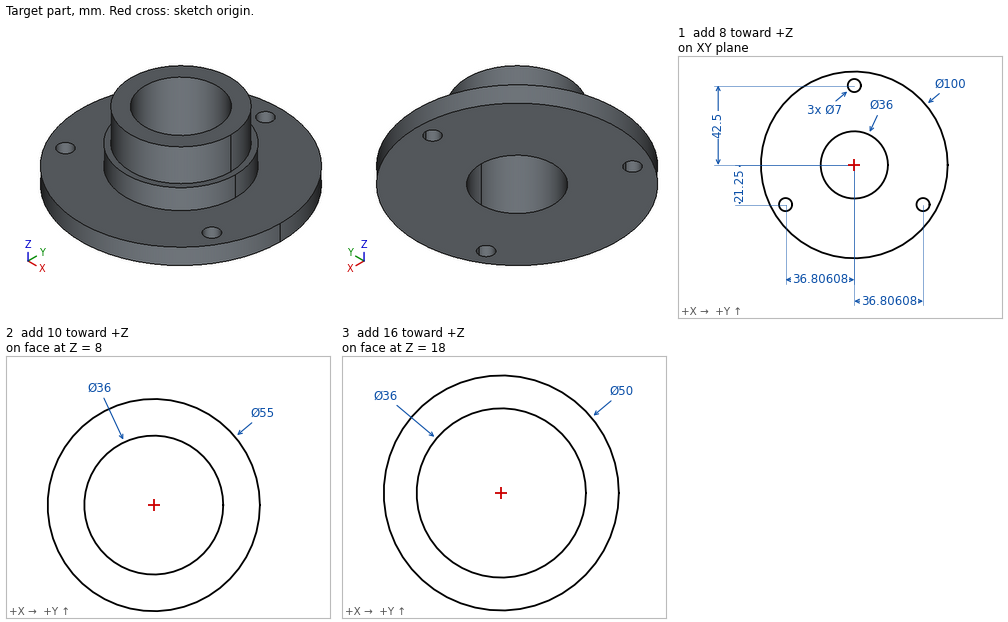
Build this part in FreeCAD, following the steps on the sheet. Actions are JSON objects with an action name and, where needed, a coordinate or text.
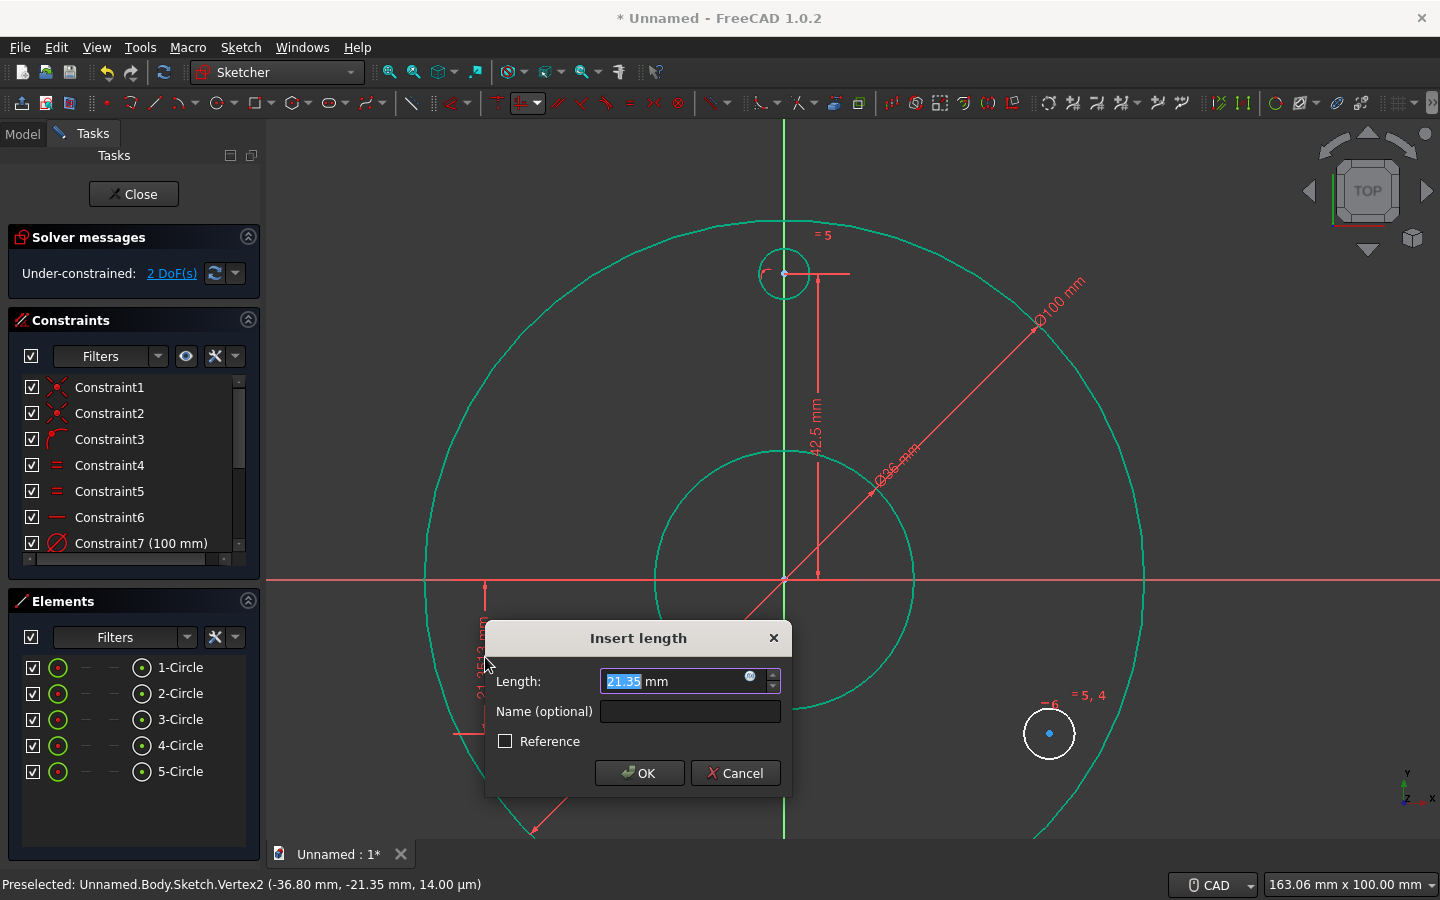
{"action": "type", "text": "21.25"}
{"action": "key", "text": "Return"}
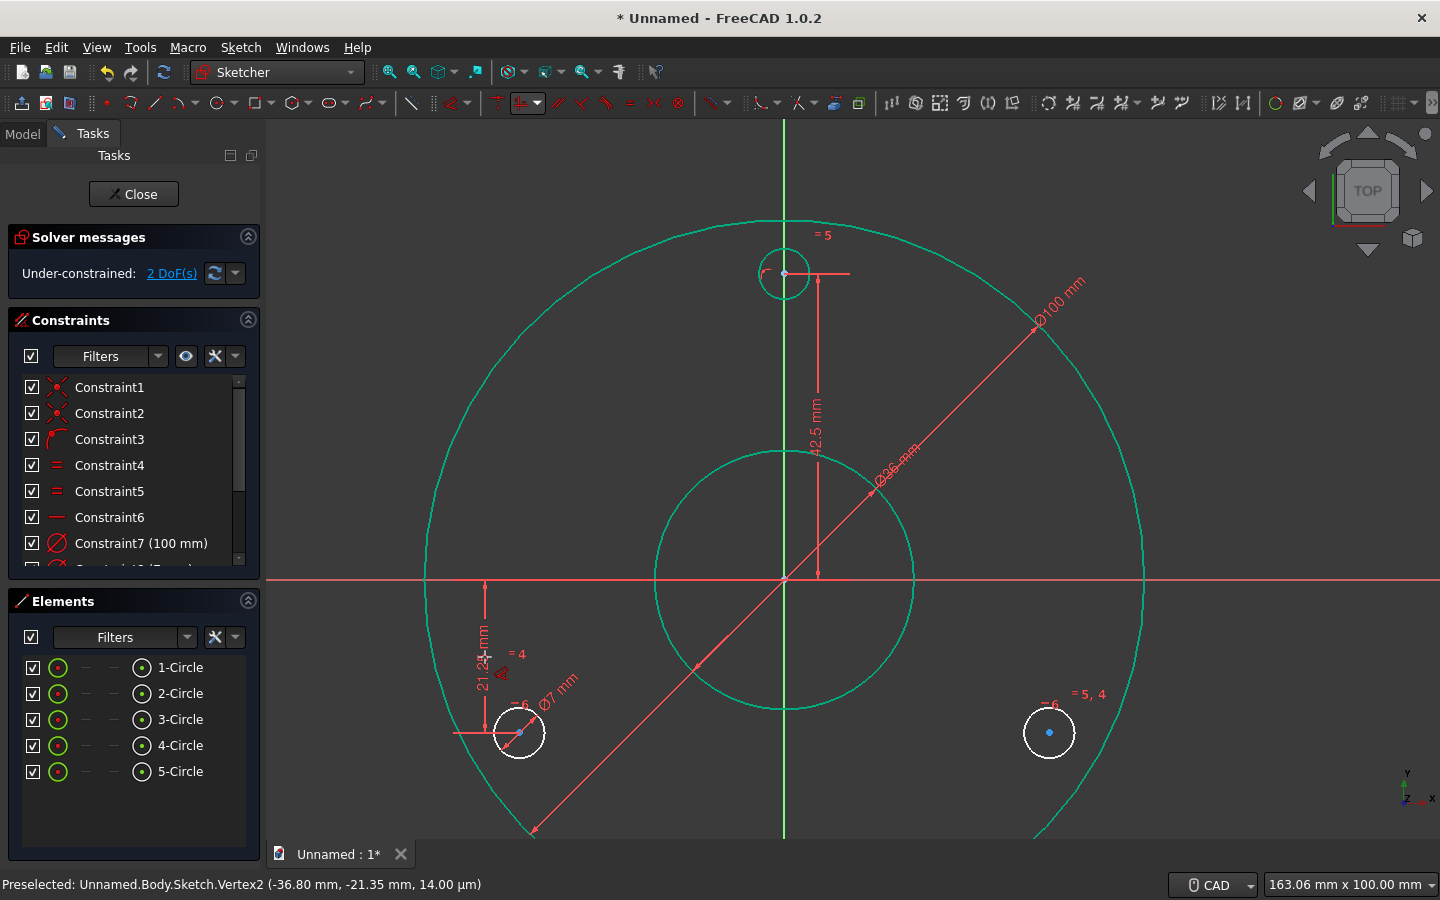
{"action": "left_click", "coordinate": [519, 733]}
{"action": "left_click", "coordinate": [652, 767]}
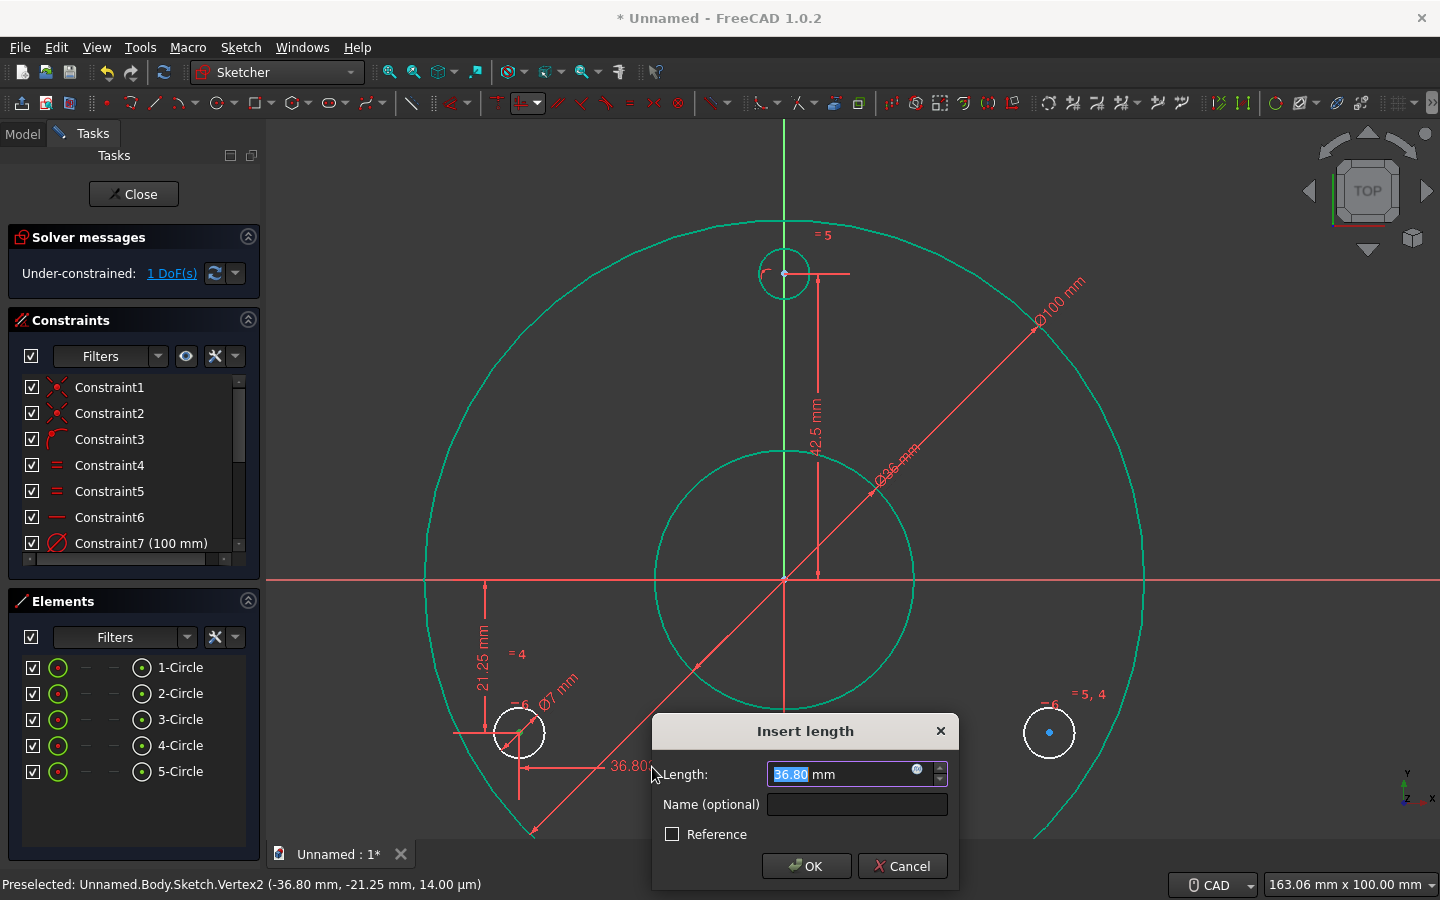
{"action": "type", "text": "36.80608"}
{"action": "key", "text": "Return"}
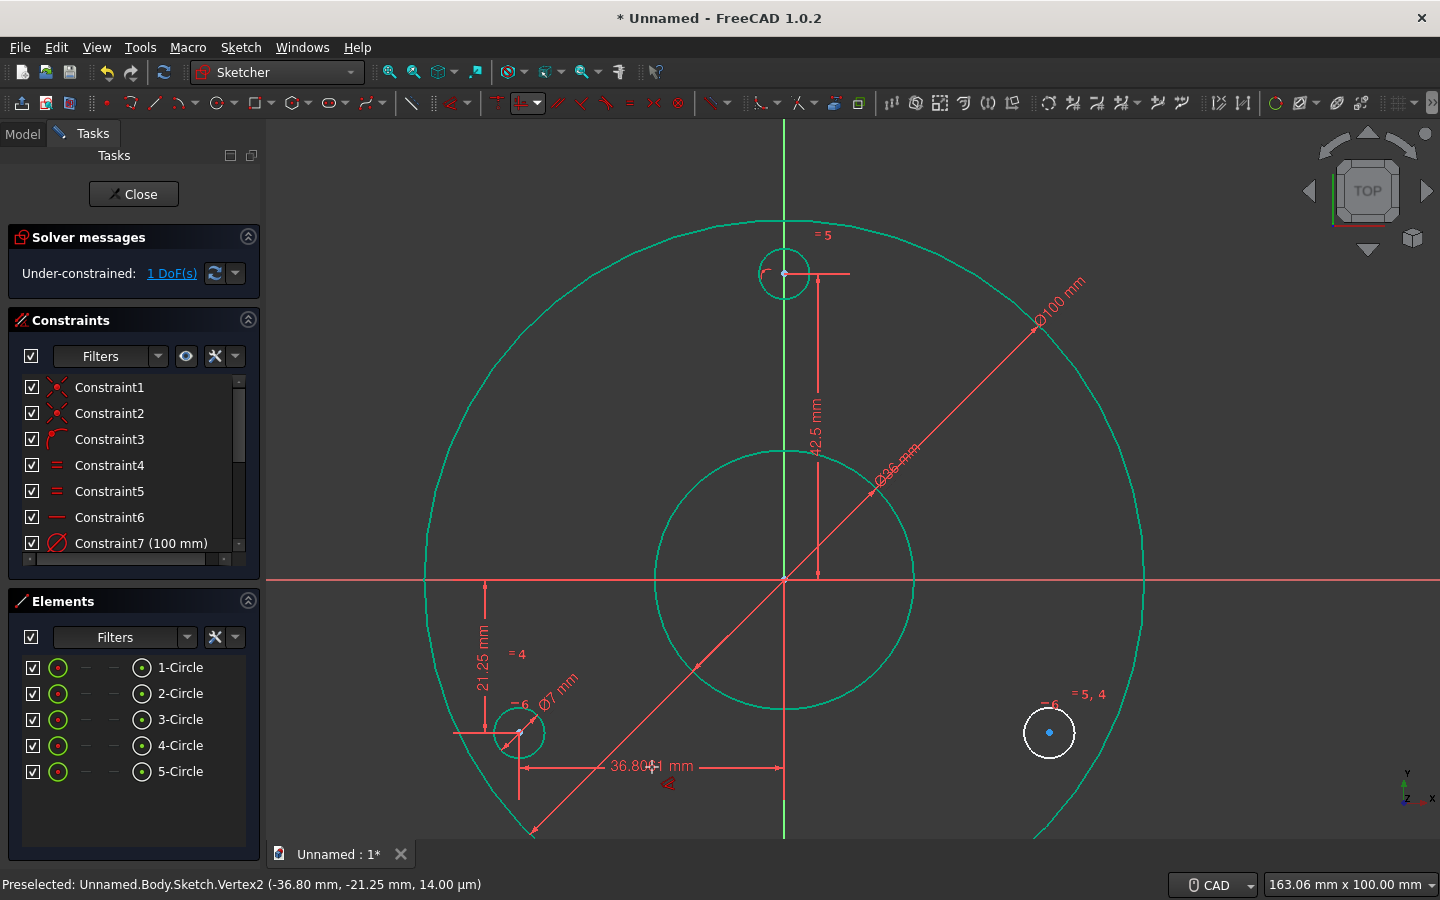
{"action": "left_click", "coordinate": [1049, 733]}
{"action": "left_click", "coordinate": [917, 767]}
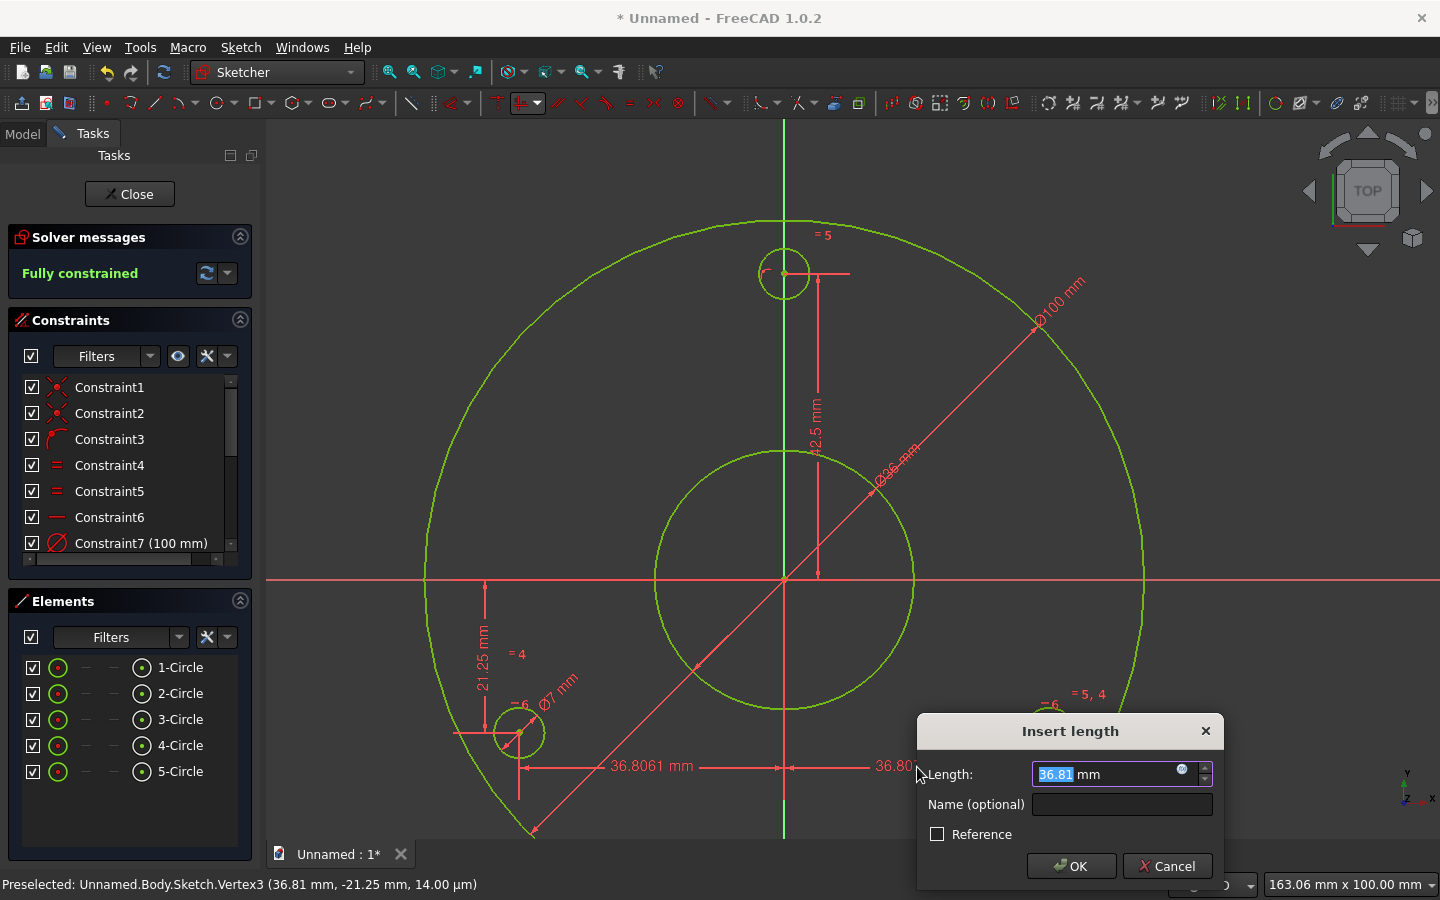
{"action": "type", "text": "36.80608"}
{"action": "key", "text": "Return"}
{"action": "key", "text": "Escape"}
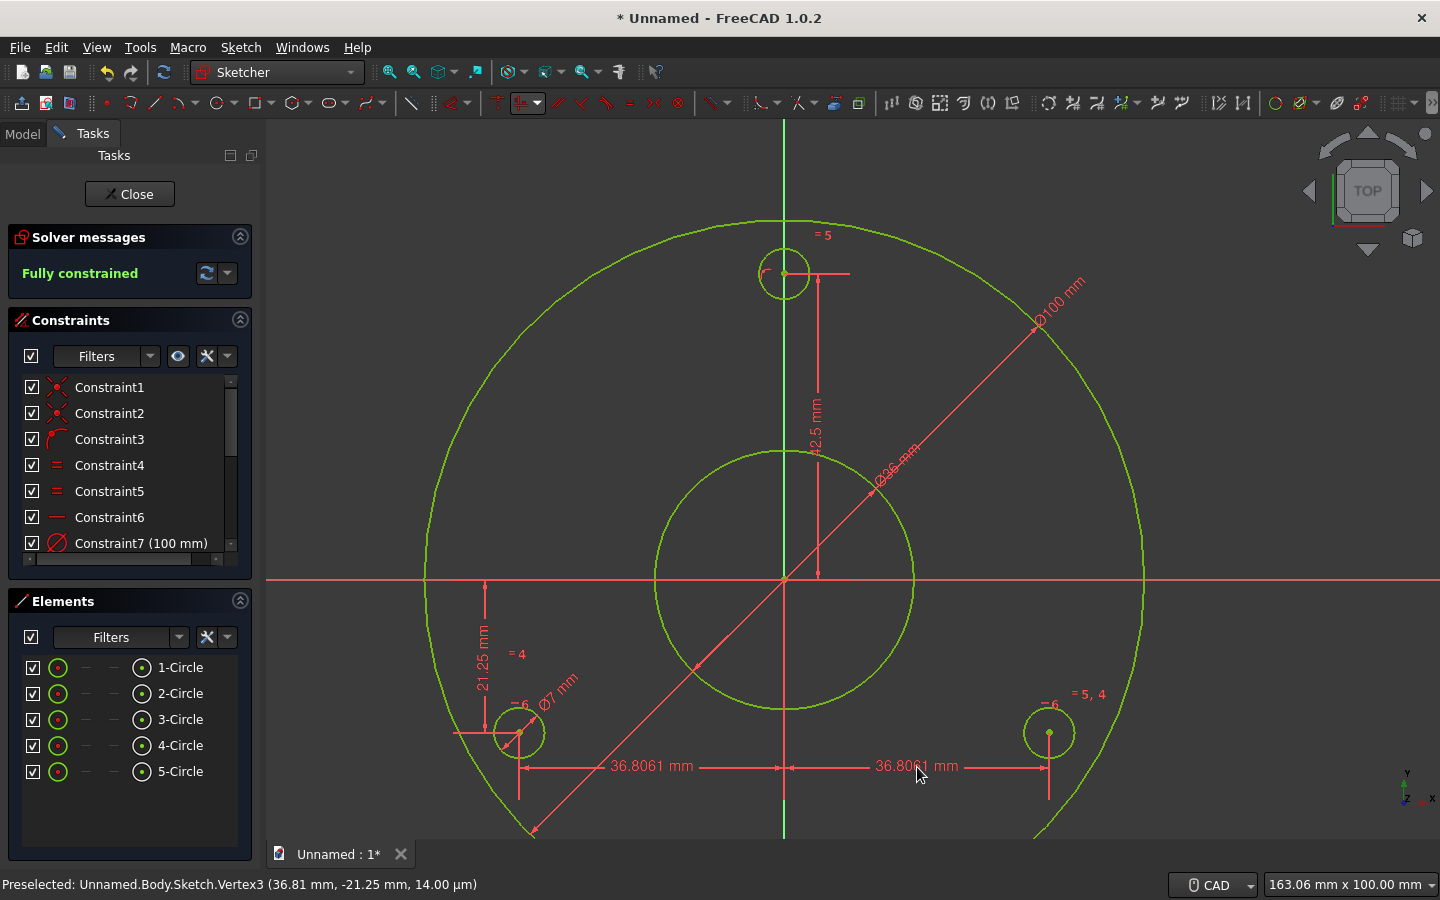
{"action": "left_click", "coordinate": [130, 194]}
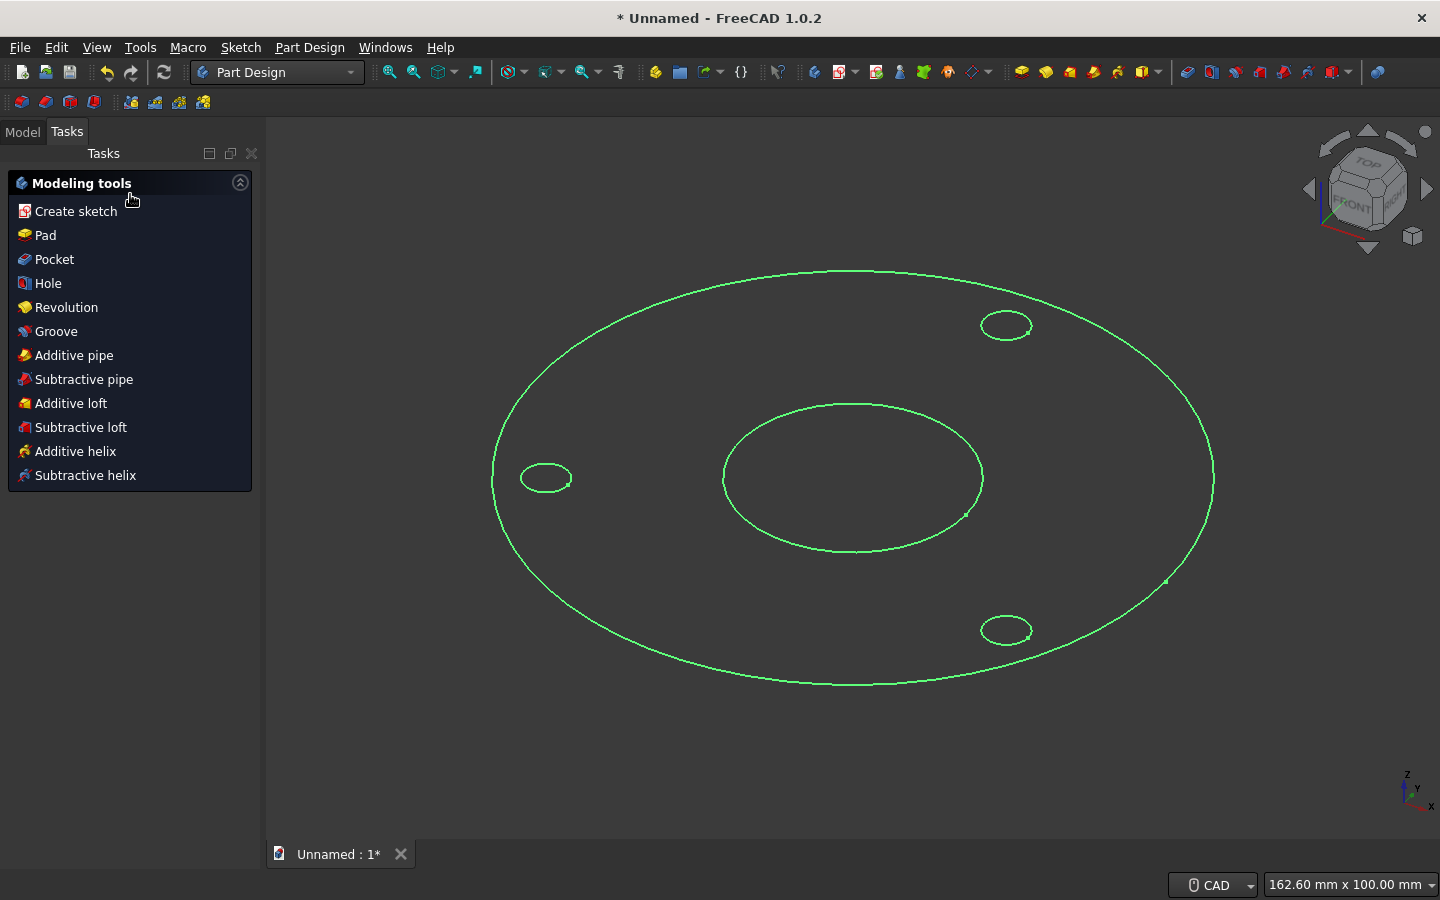
{"action": "left_click", "coordinate": [1022, 72]}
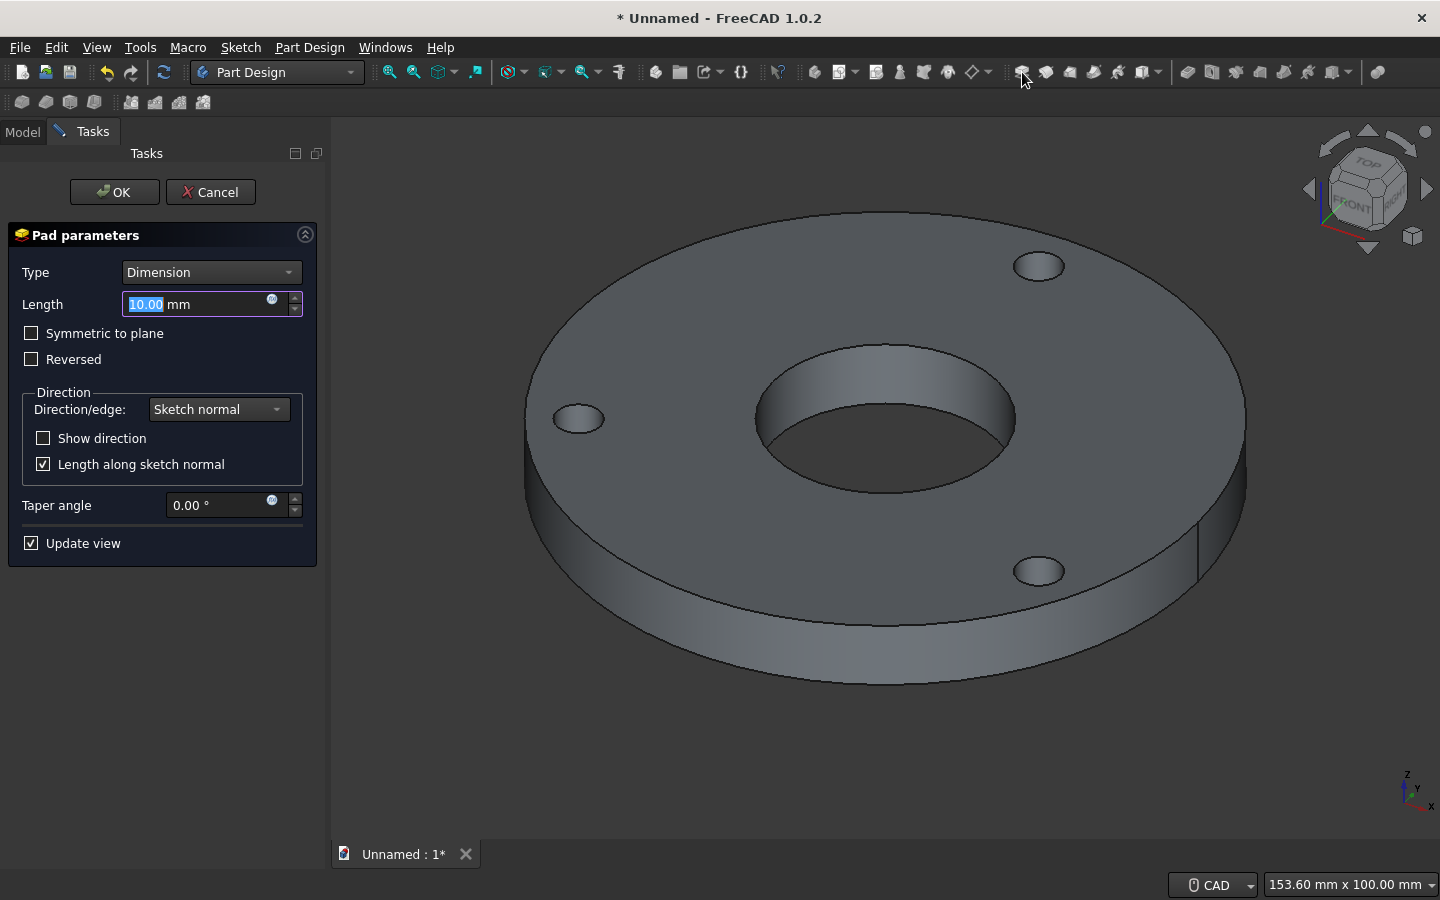
{"action": "type", "text": "8"}
{"action": "key", "text": "Tab"}